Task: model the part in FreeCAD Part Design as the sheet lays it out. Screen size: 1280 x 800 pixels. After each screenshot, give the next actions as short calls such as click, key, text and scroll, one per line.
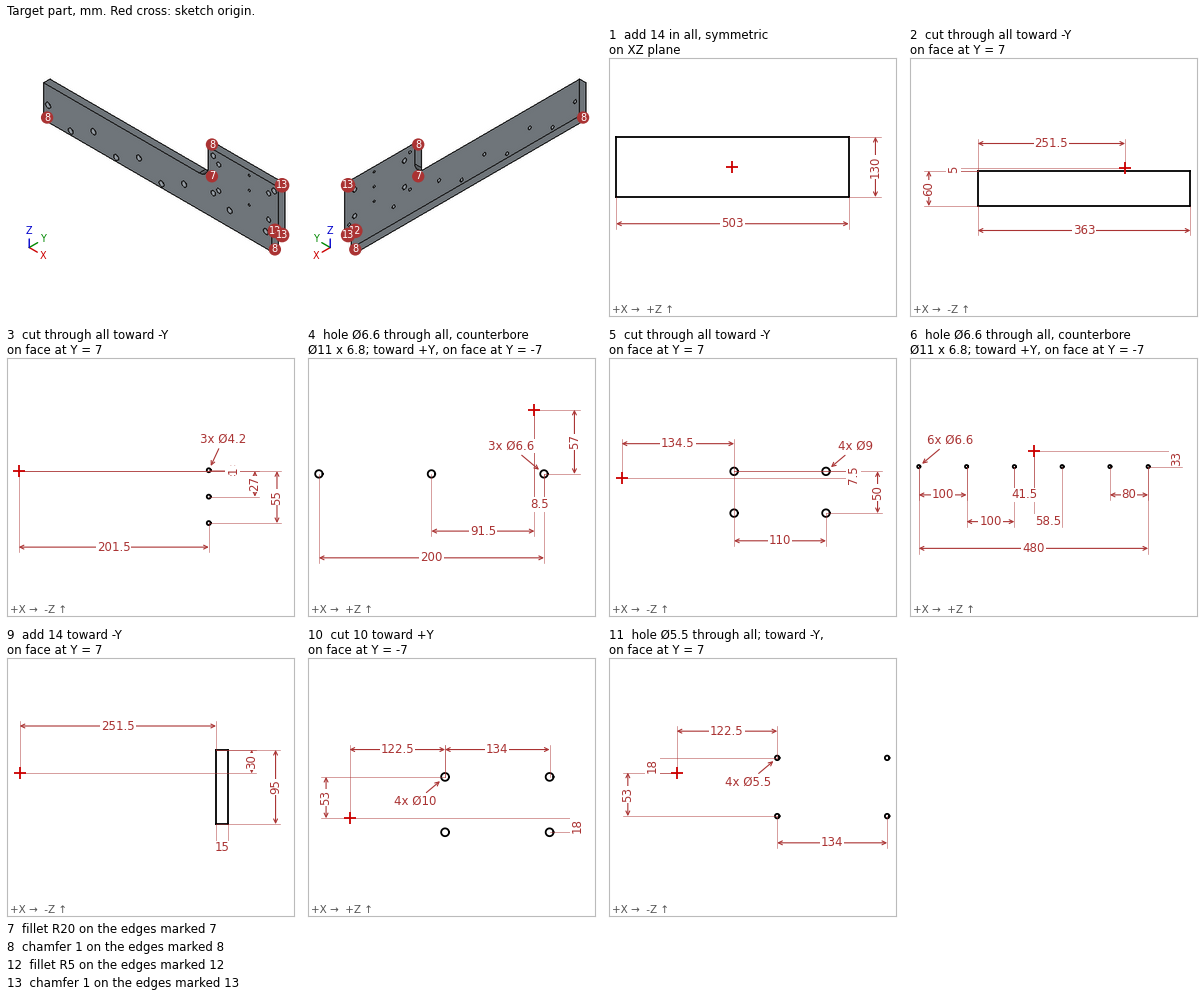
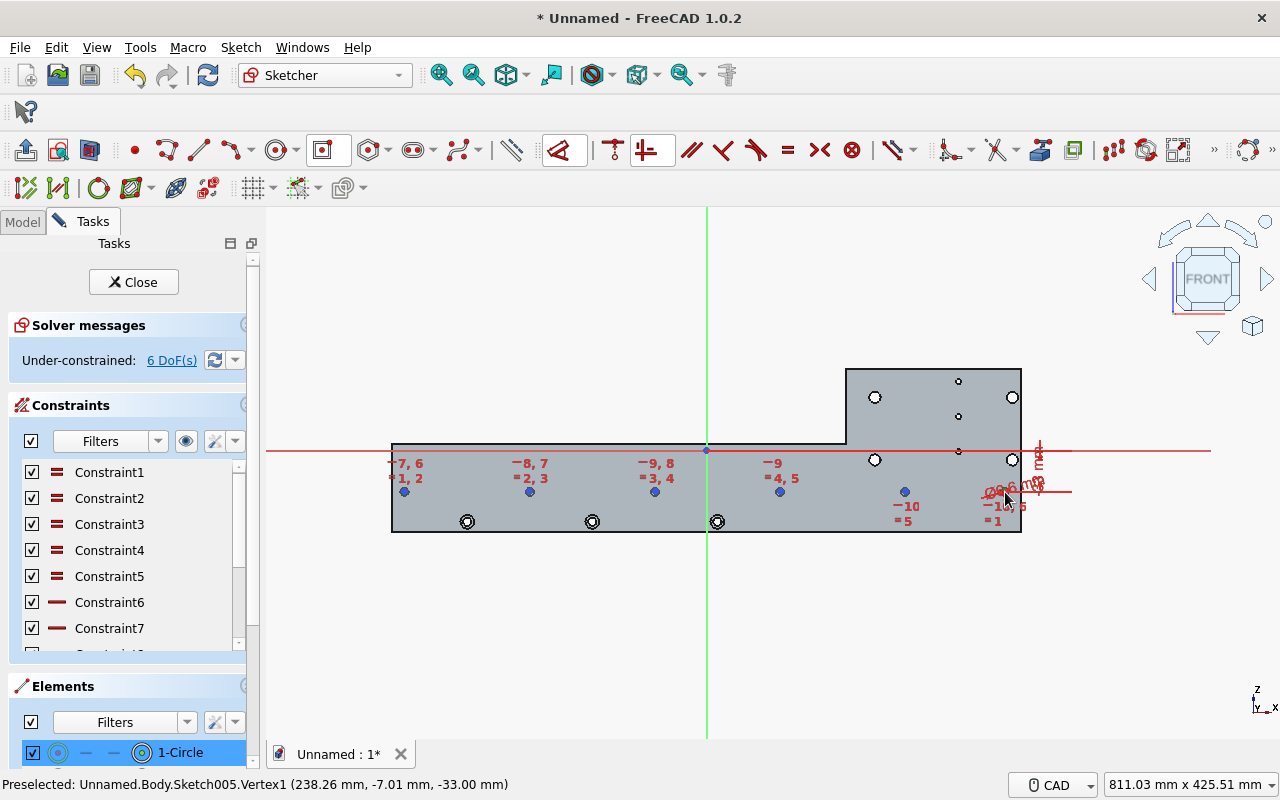
click(905, 492)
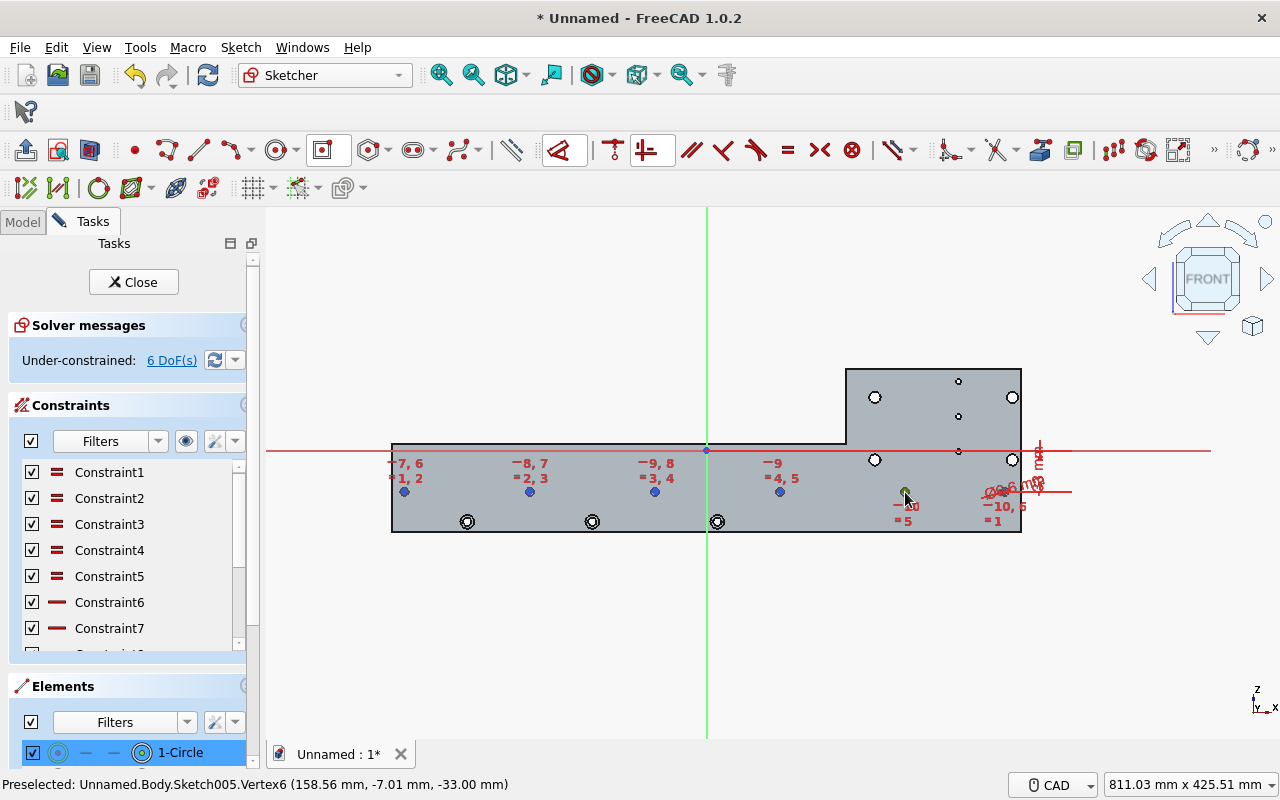
click(582, 150)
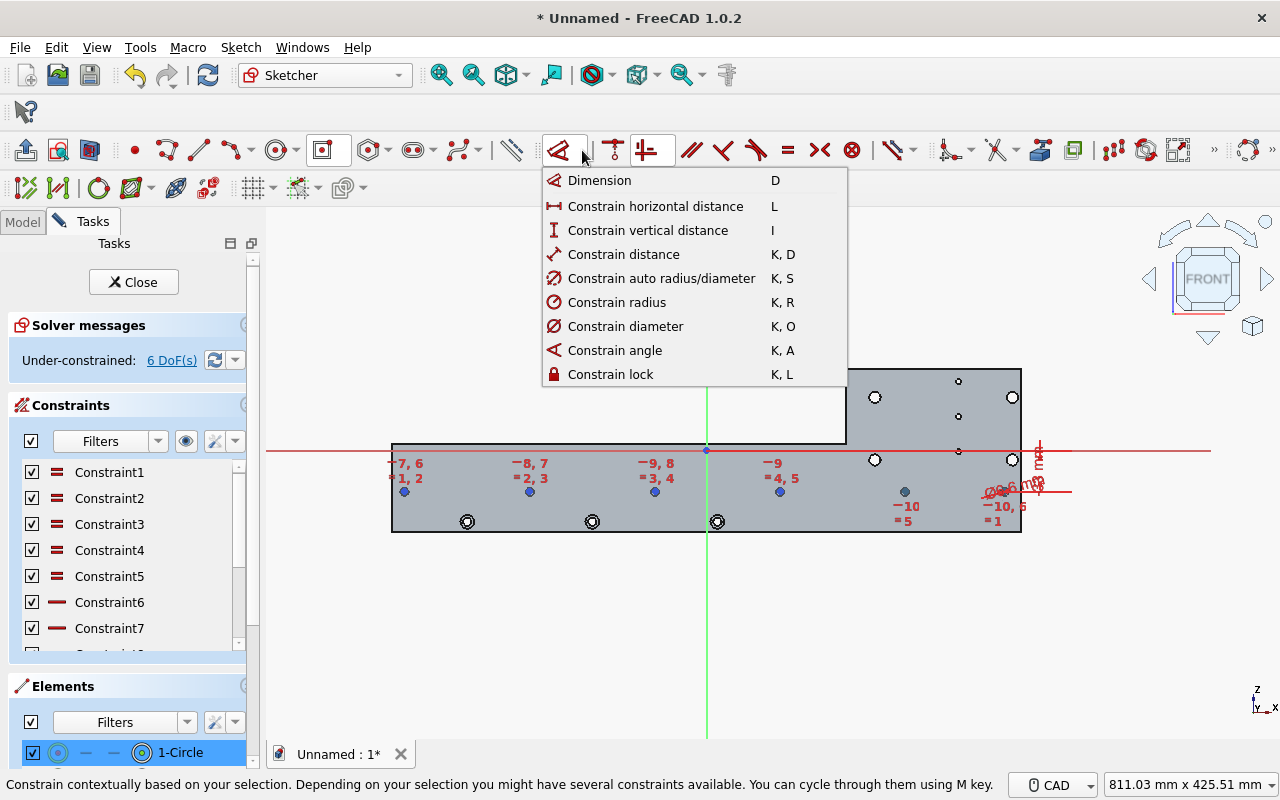
click(695, 206)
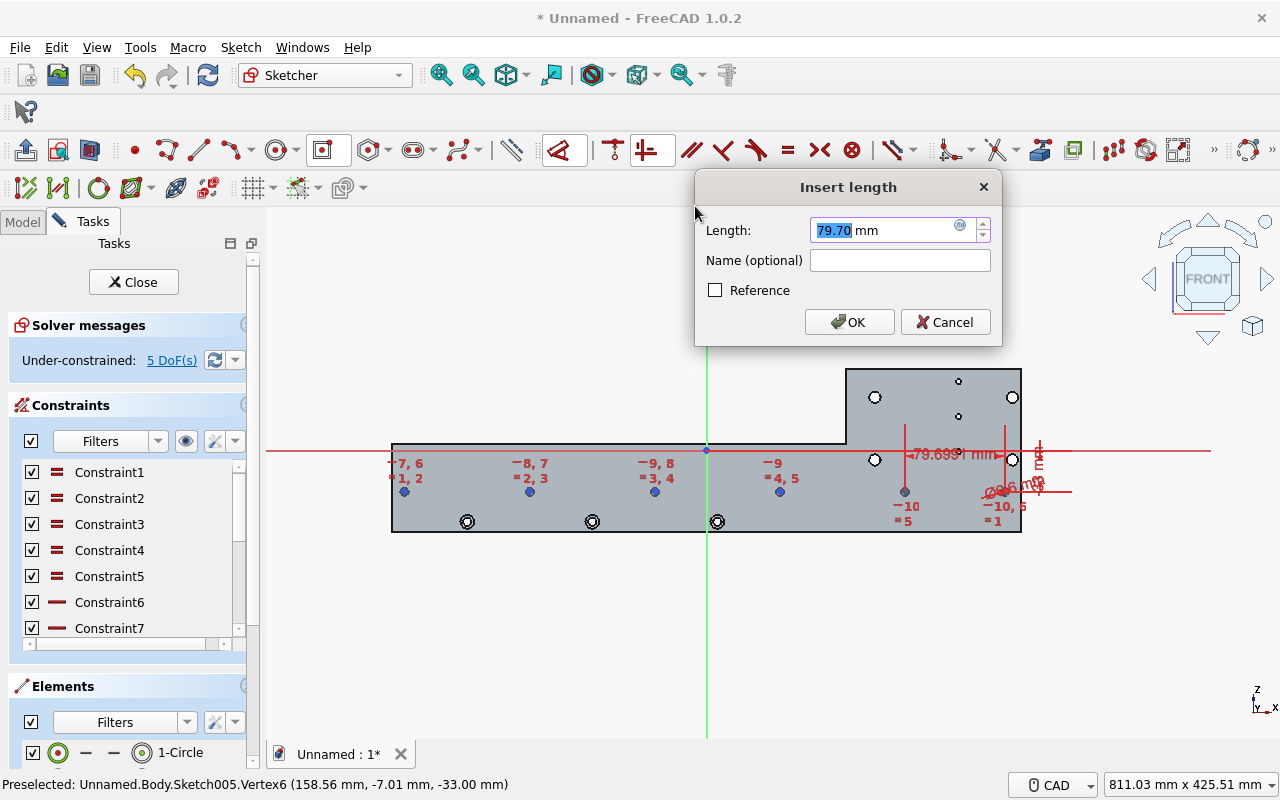
text(80)
key(Return)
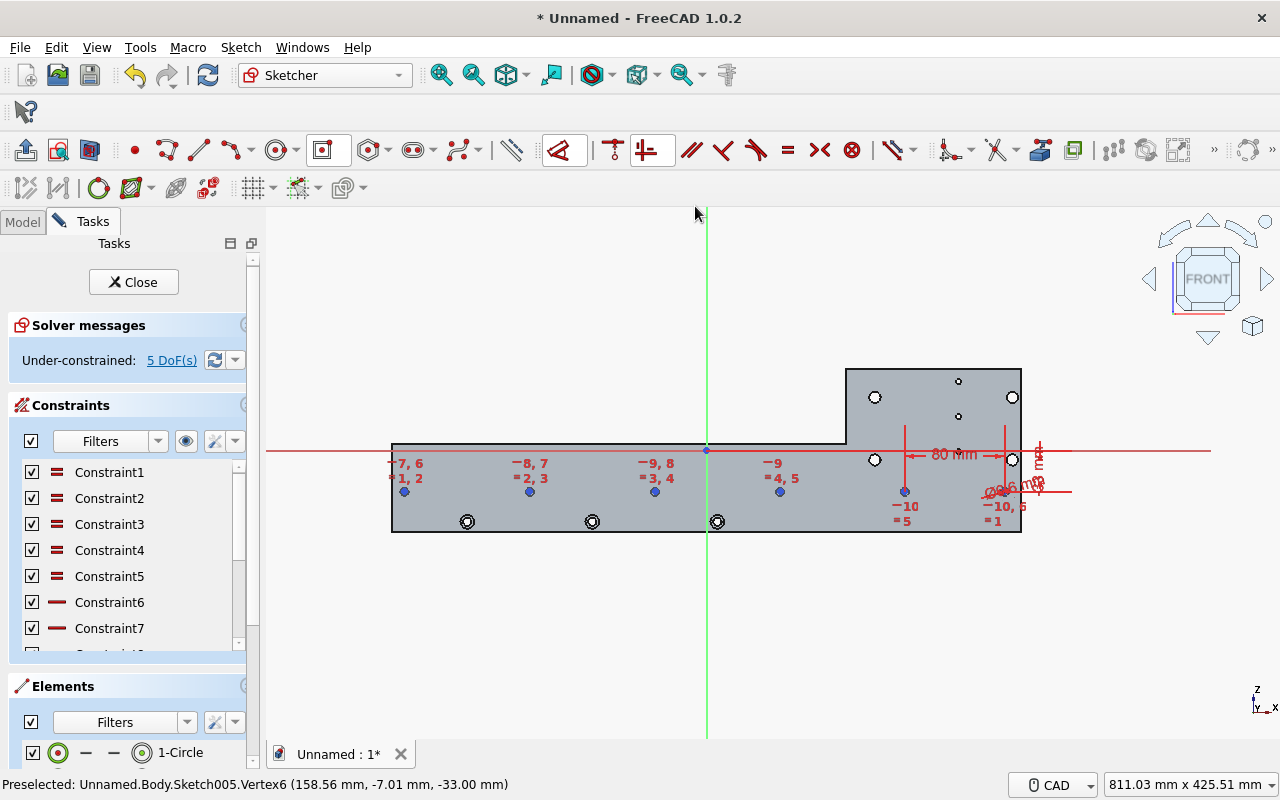
click(655, 492)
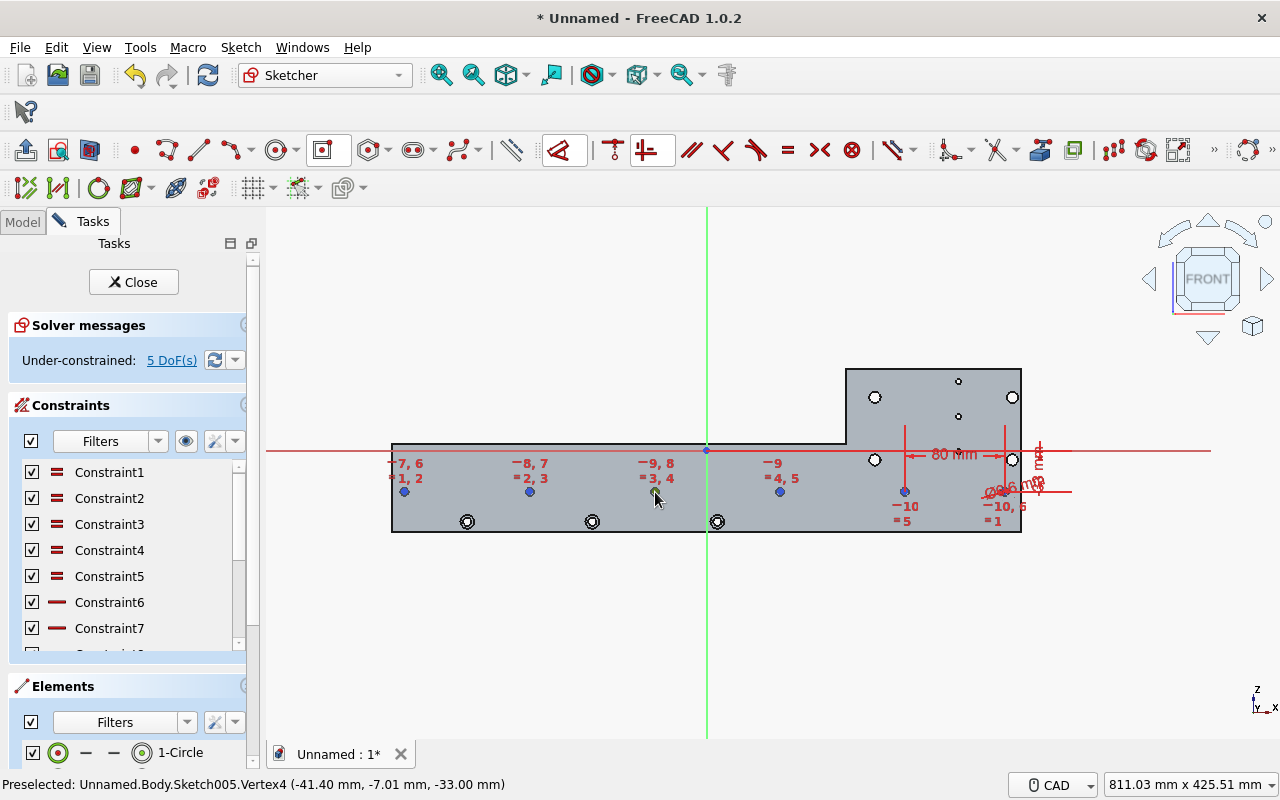
key(l)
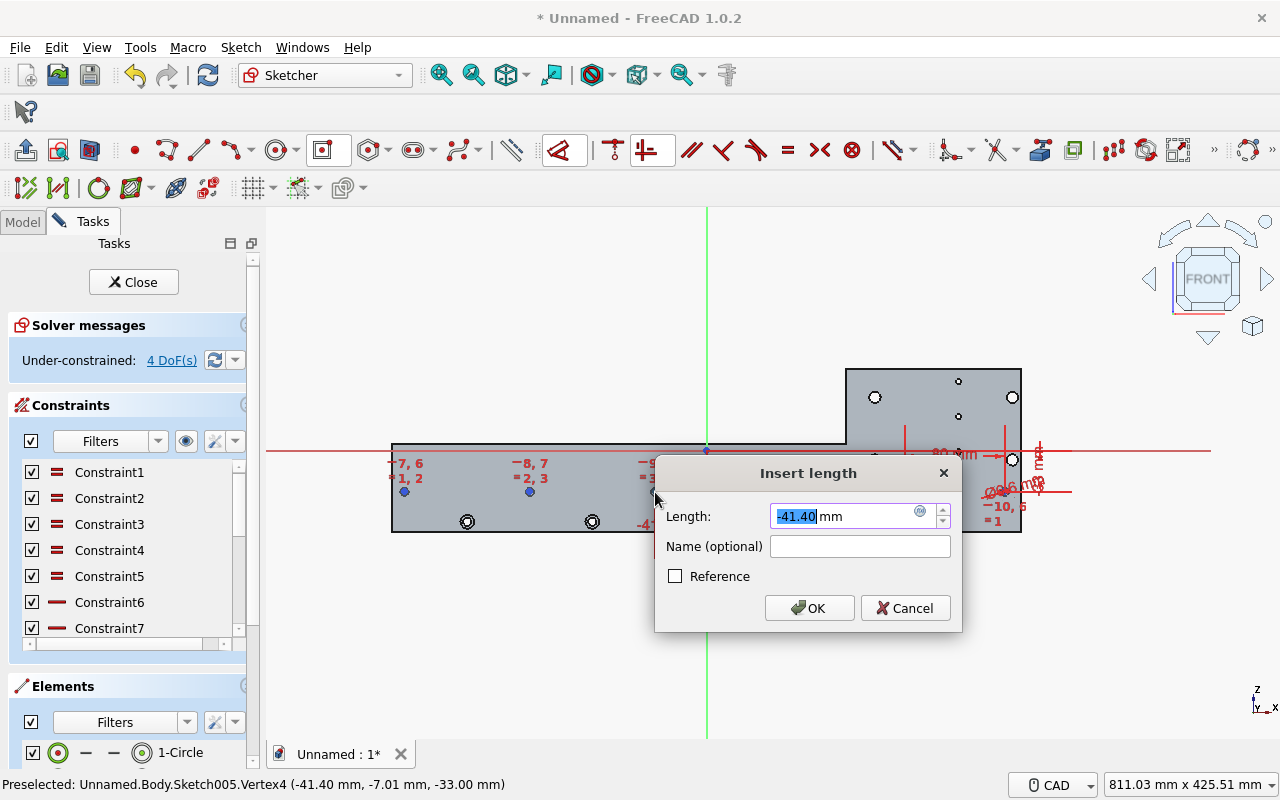
text(-41.5)
key(Return)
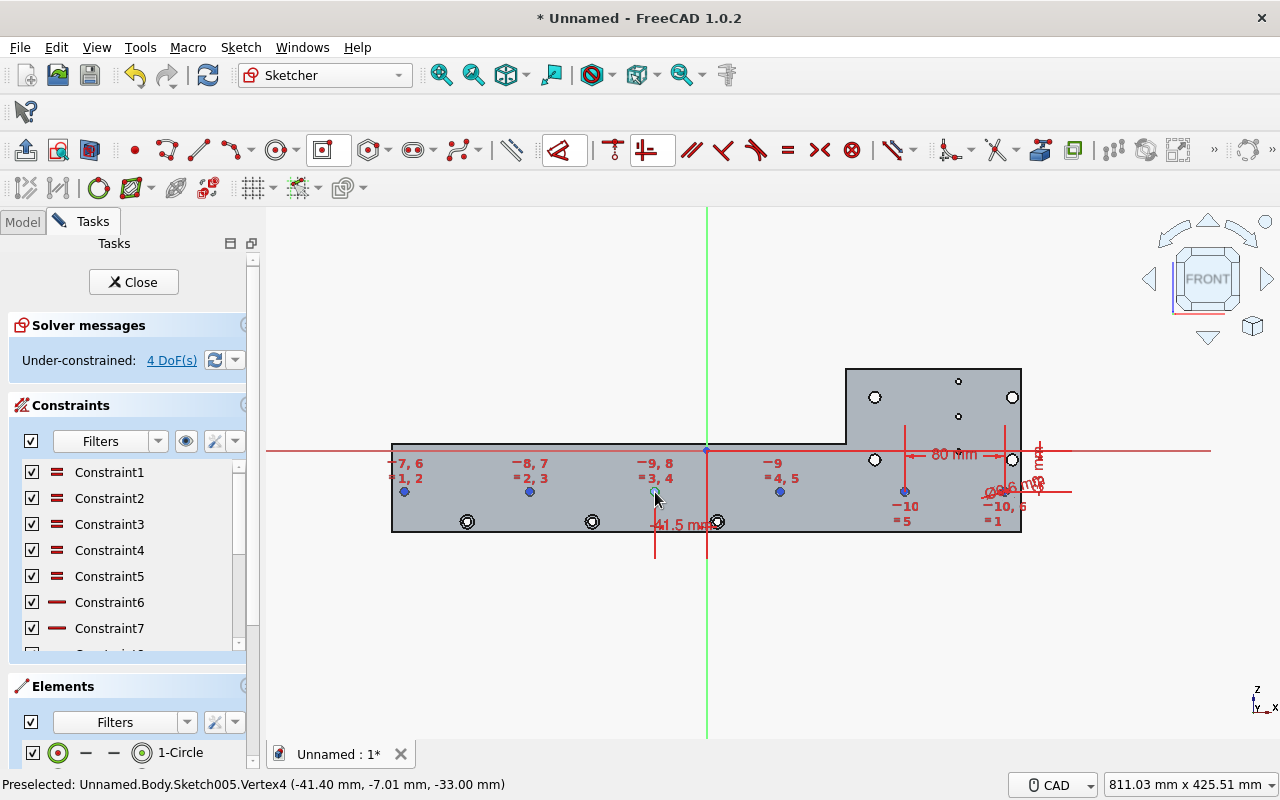
click(780, 492)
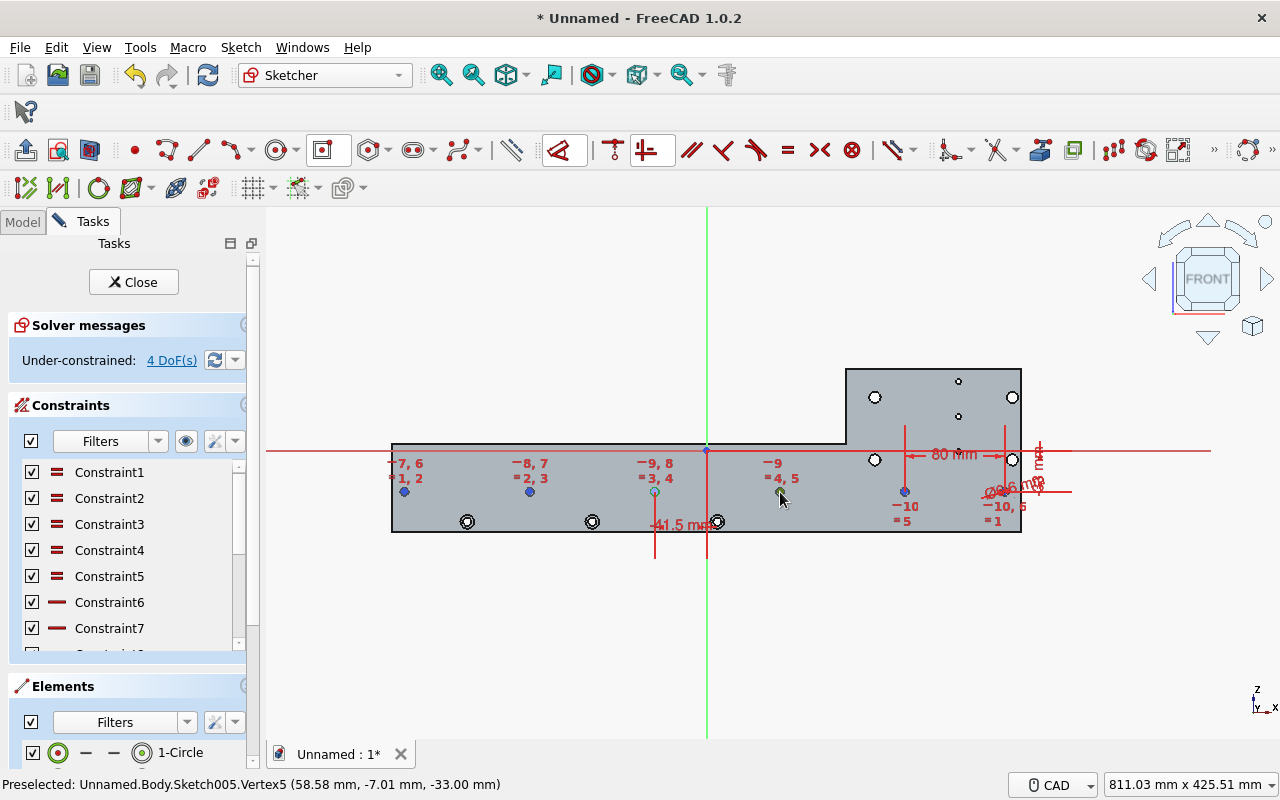
key(l)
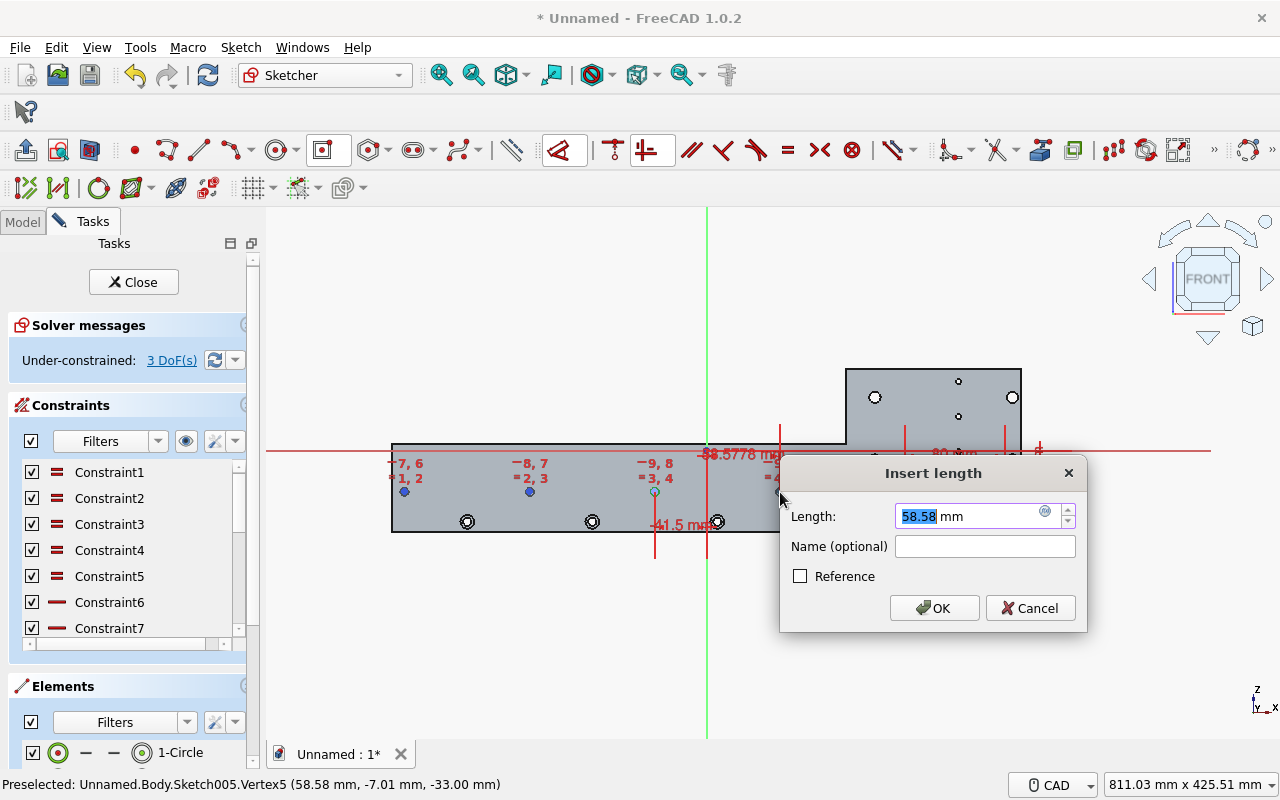
text(58.5)
key(Return)